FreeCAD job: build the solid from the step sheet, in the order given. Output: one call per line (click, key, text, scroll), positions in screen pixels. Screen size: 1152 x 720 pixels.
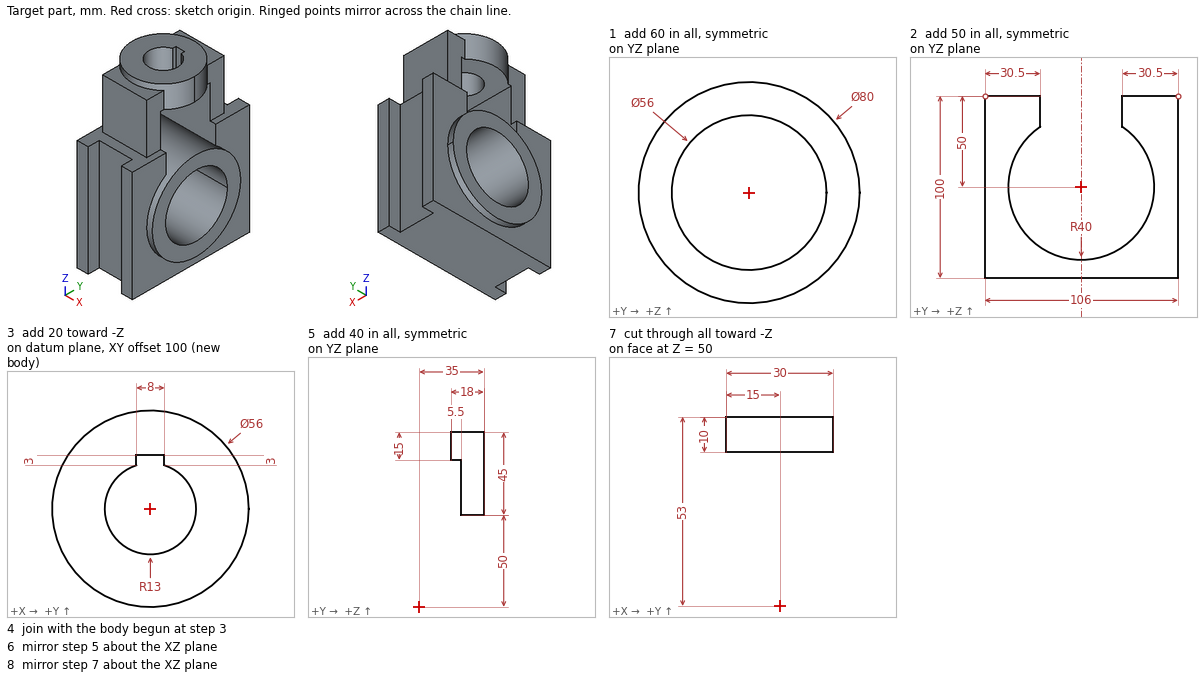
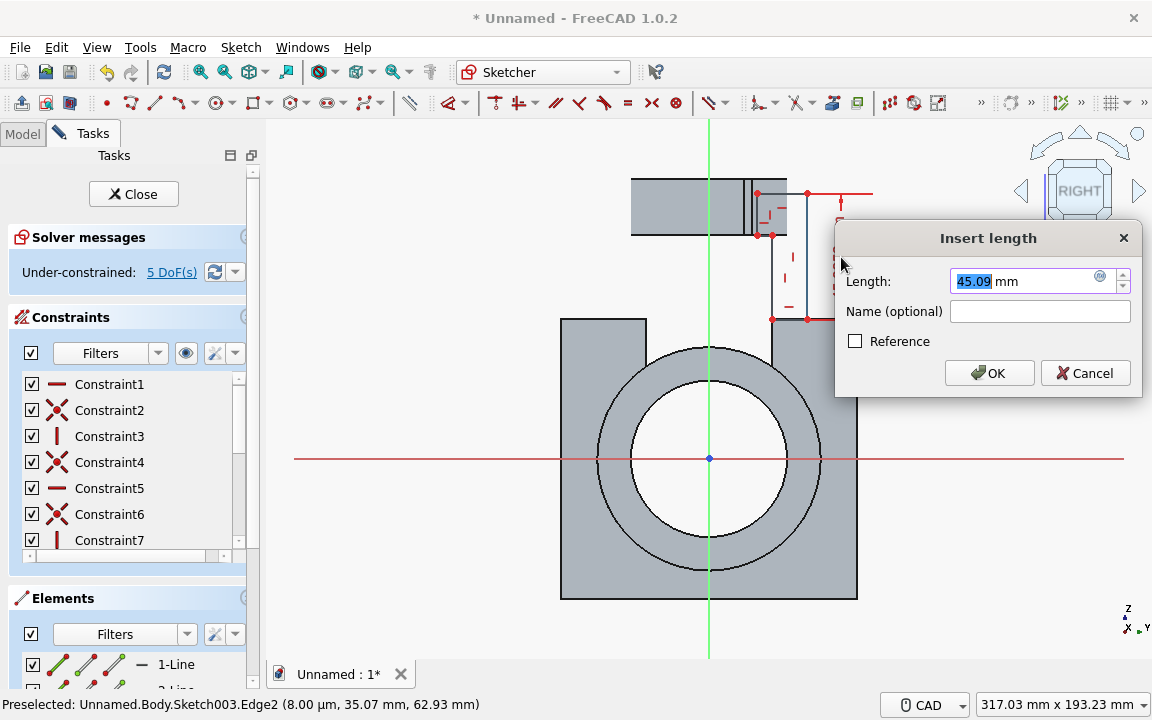
text(45)
key(Return)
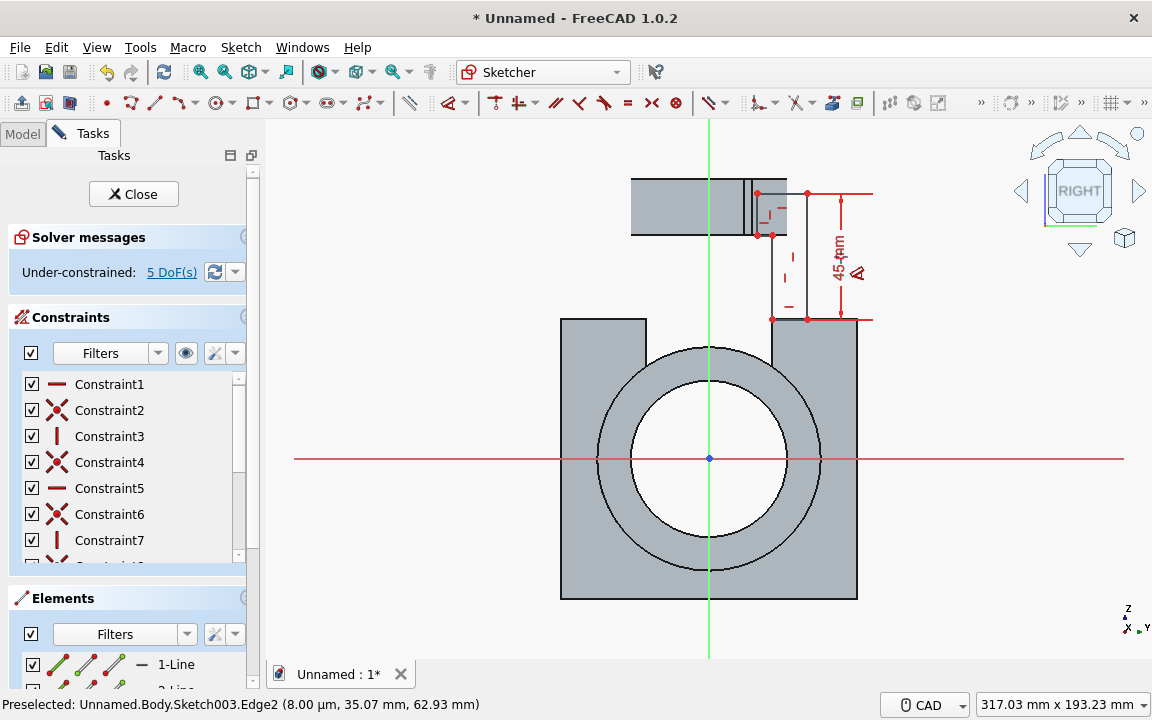
click(792, 194)
click(782, 160)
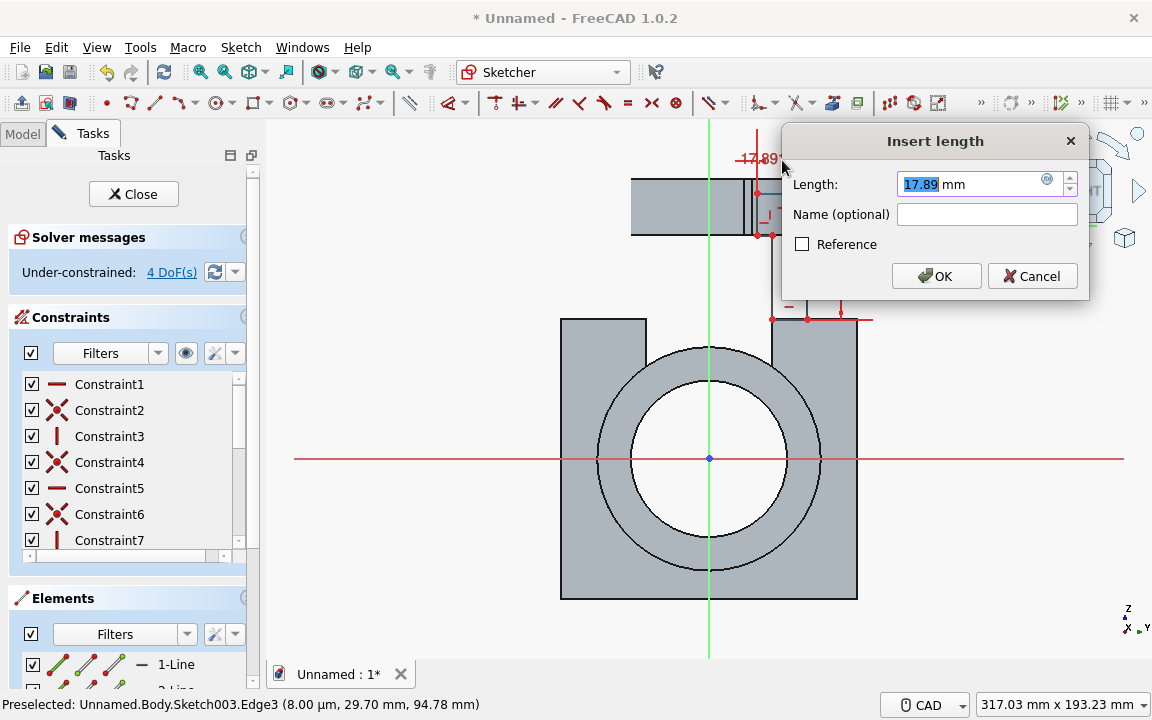
text(18)
key(Return)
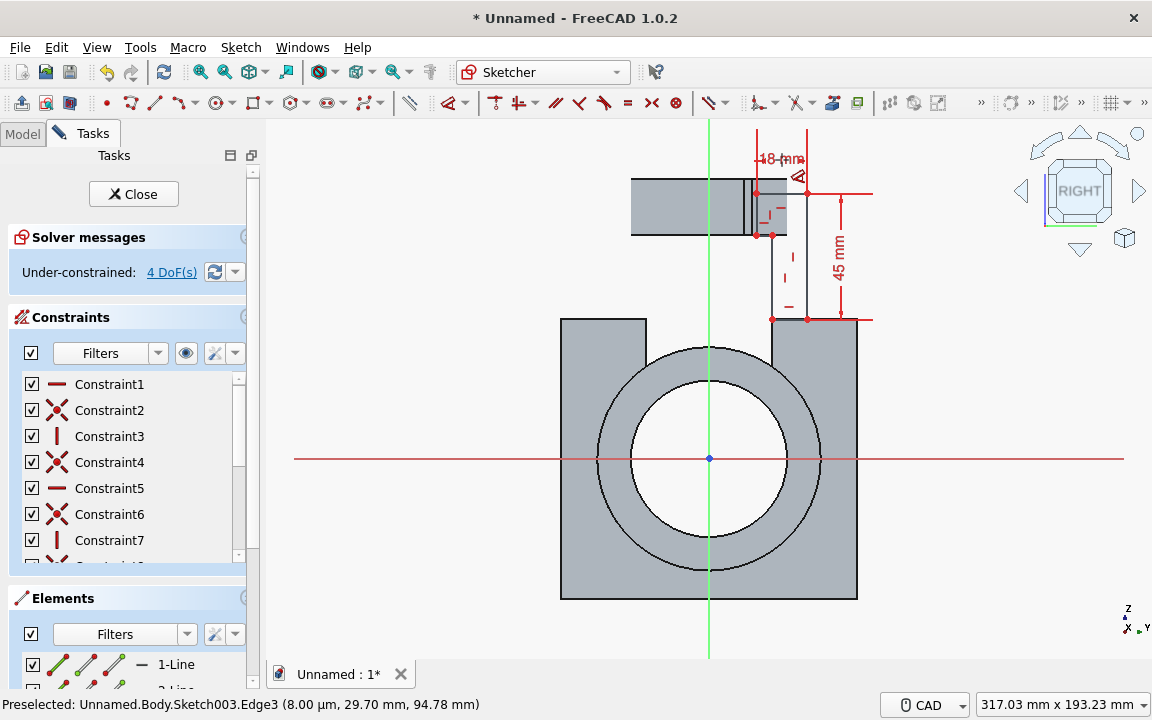
click(757, 207)
click(723, 215)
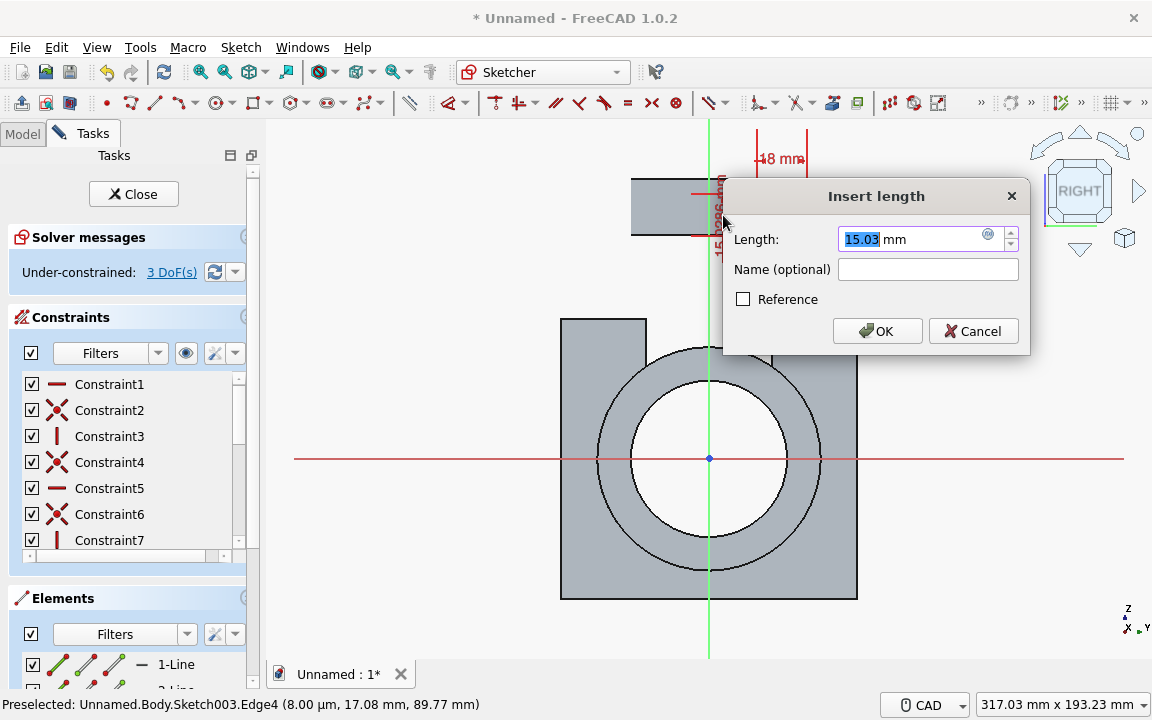
text(15)
key(Return)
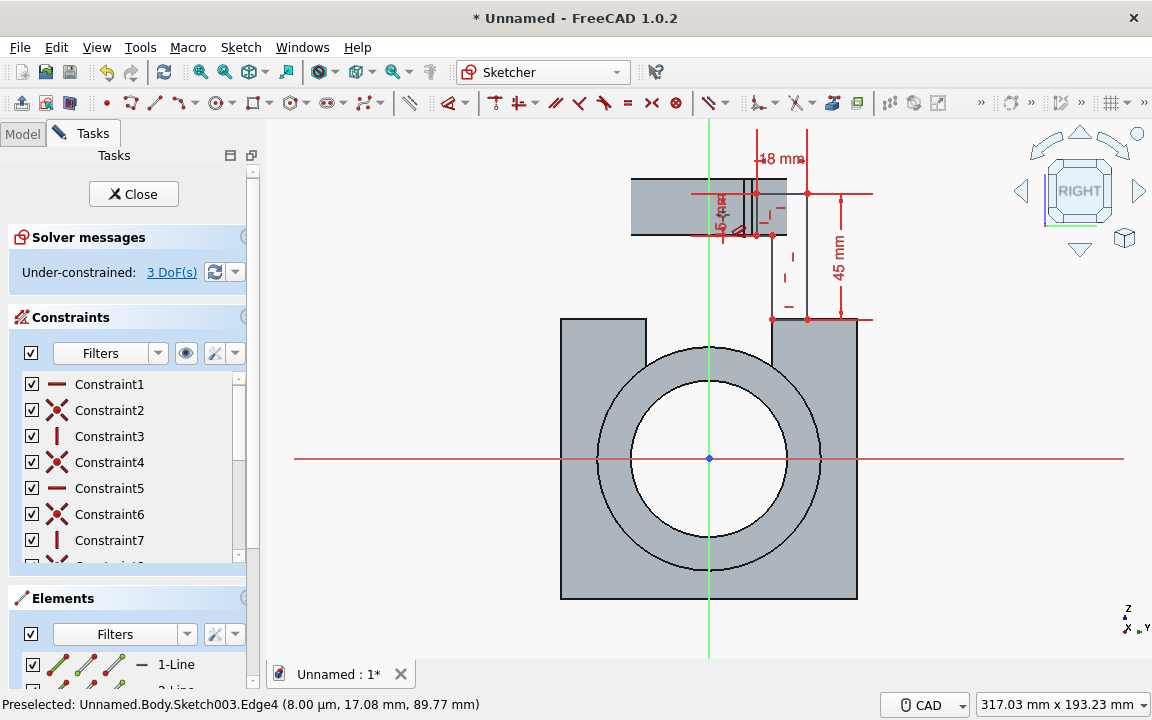
scroll(764, 236, up, 5)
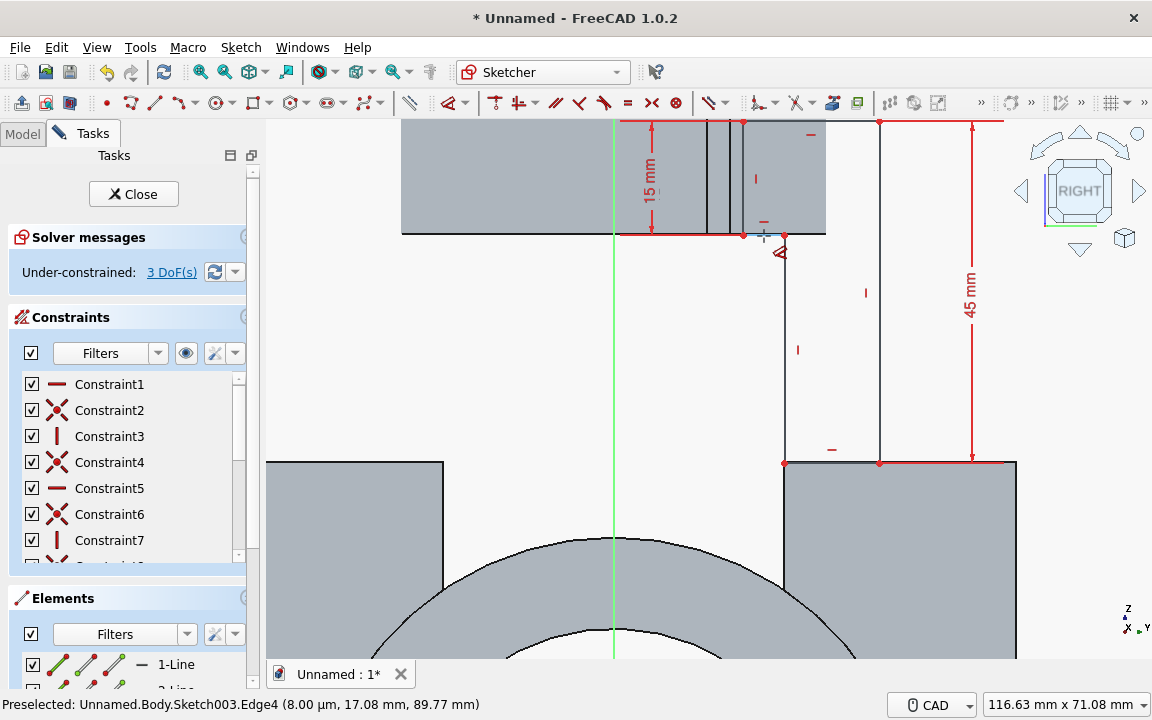
click(764, 235)
click(764, 201)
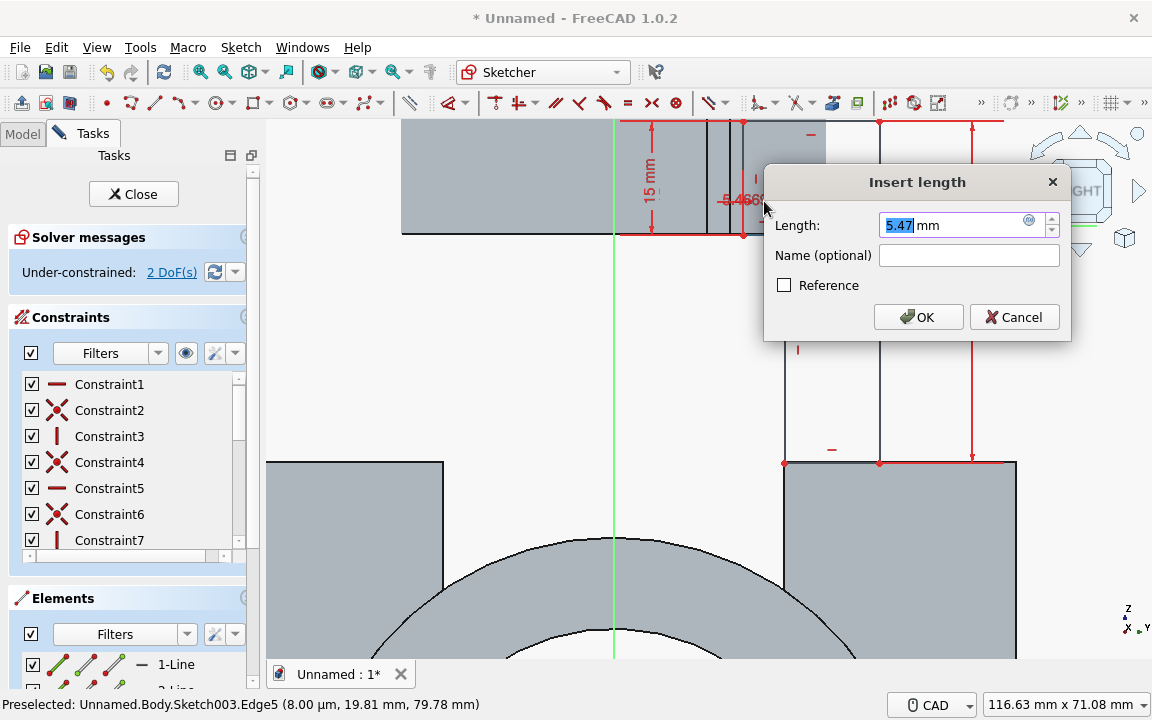
text(5.5)
key(Return)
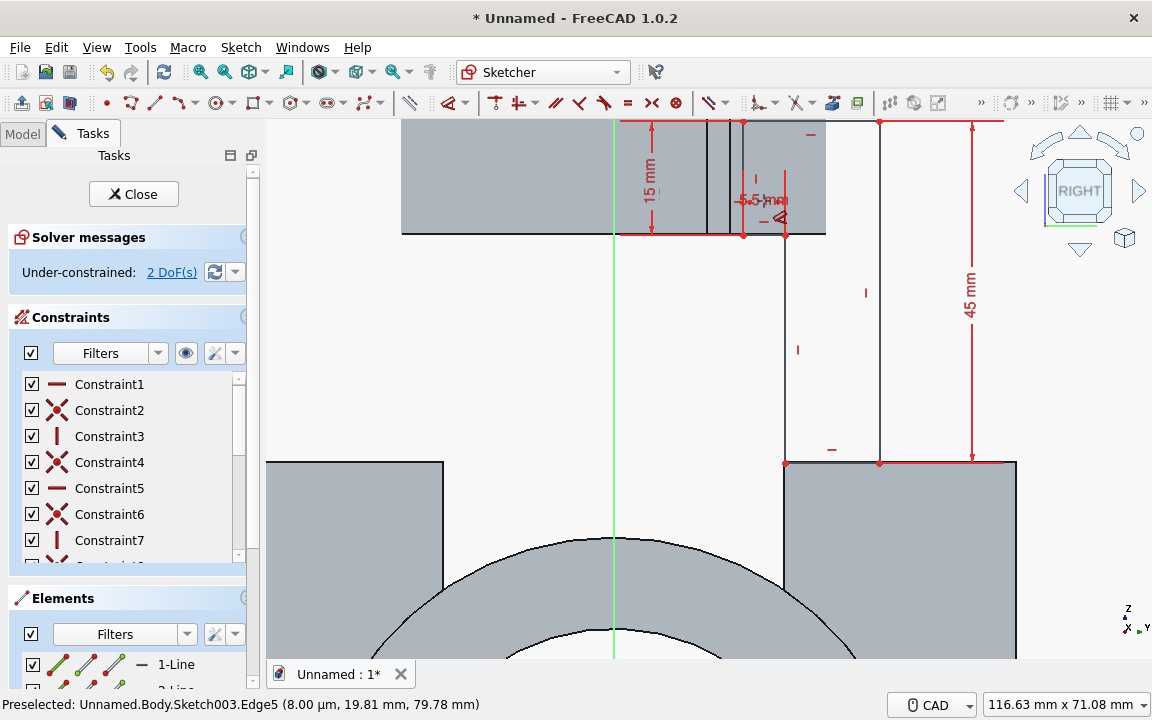
click(785, 463)
click(580, 547)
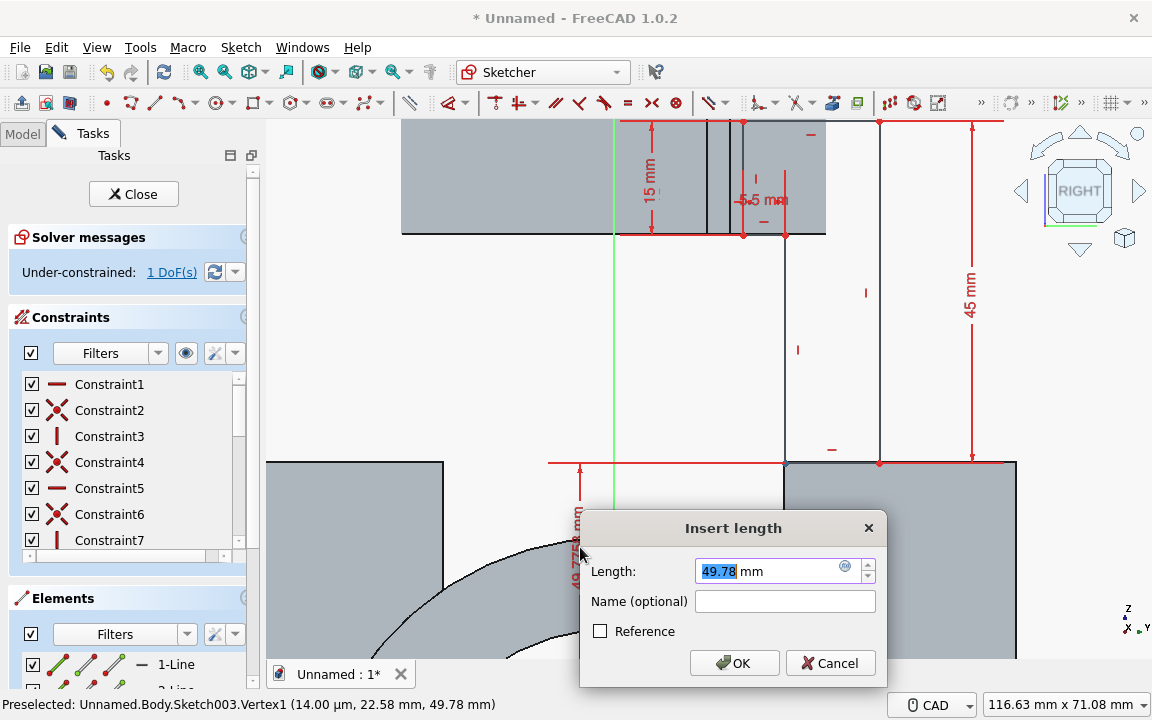
text(50)
key(Return)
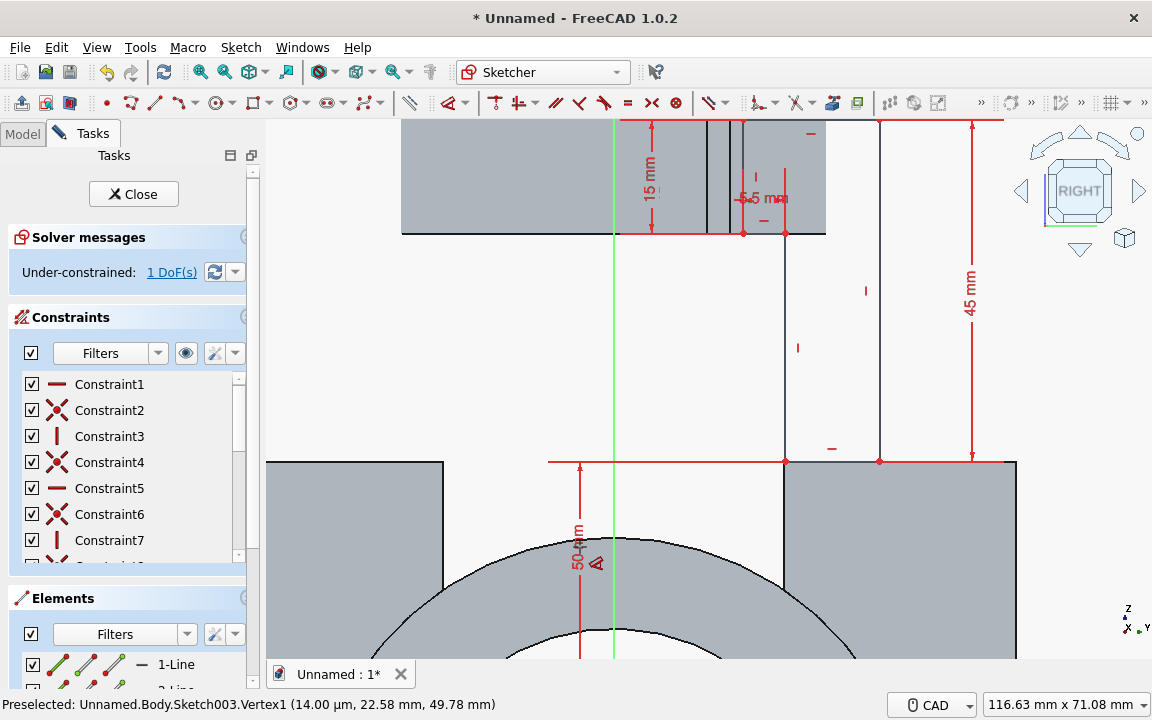
click(880, 462)
click(747, 428)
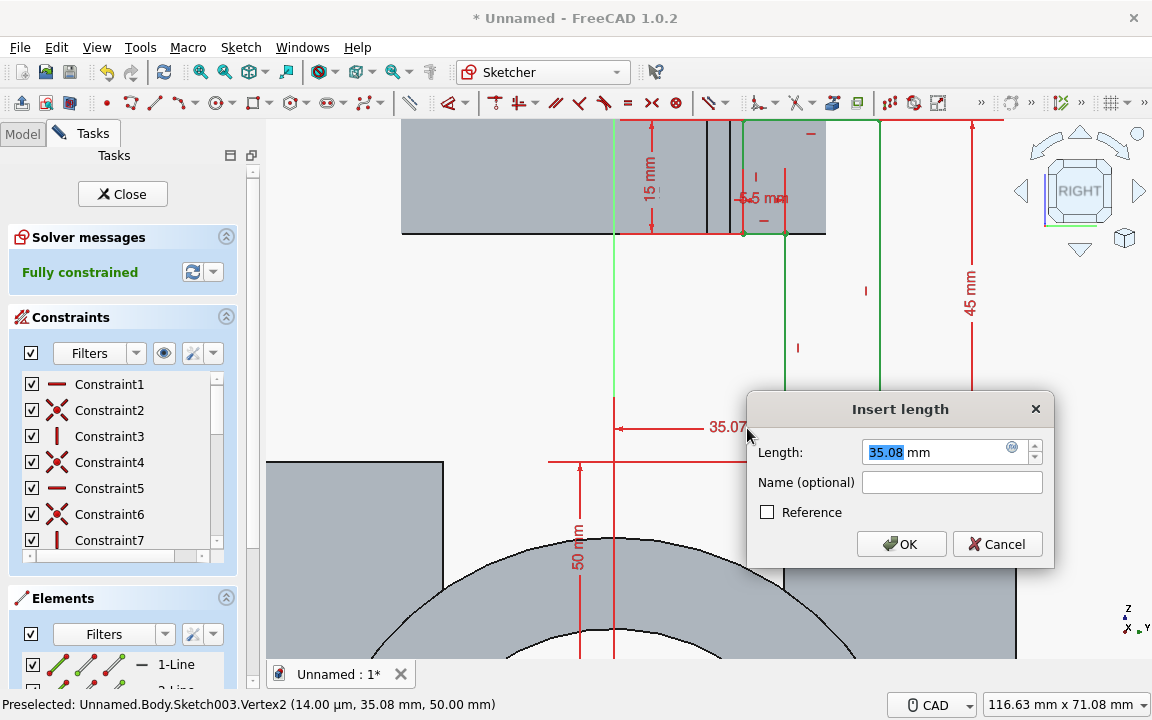
text(35)
key(Return)
key(Escape)